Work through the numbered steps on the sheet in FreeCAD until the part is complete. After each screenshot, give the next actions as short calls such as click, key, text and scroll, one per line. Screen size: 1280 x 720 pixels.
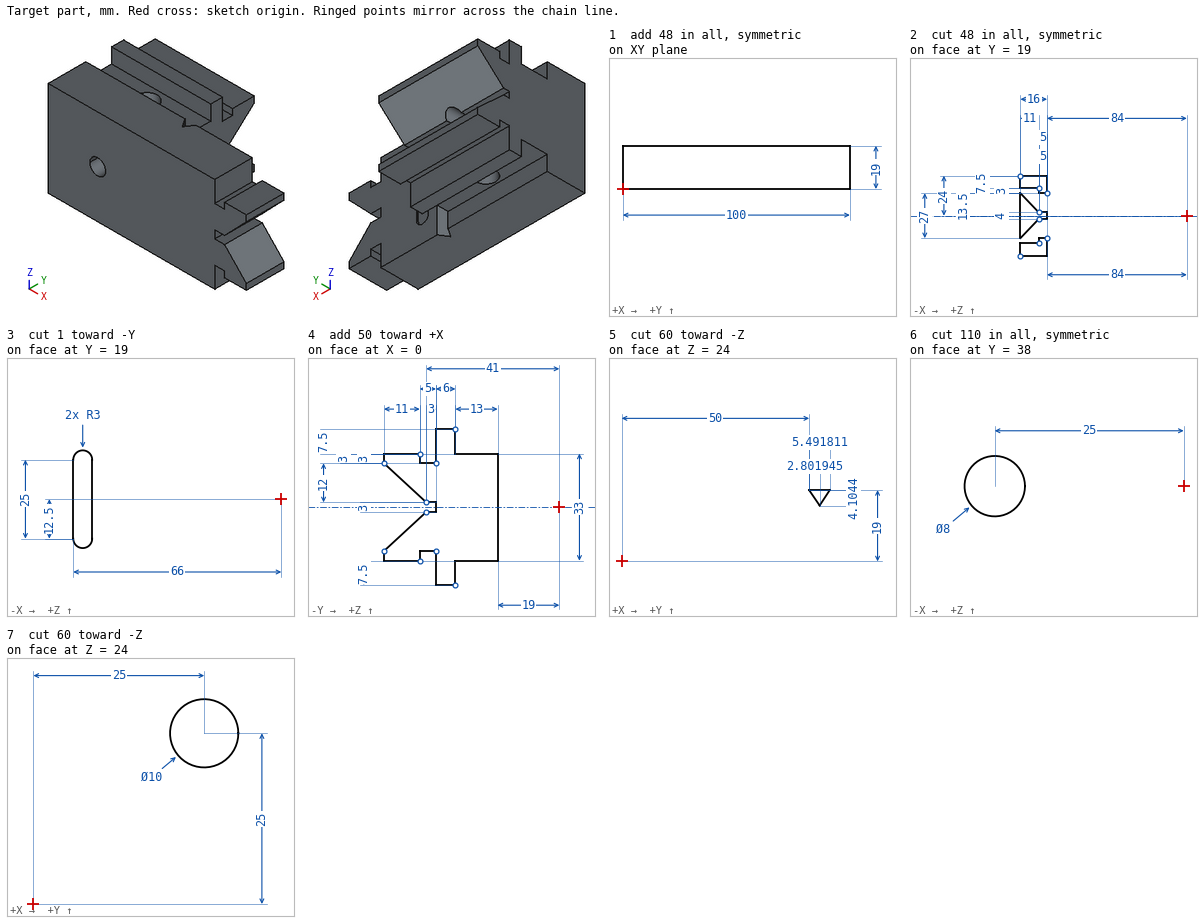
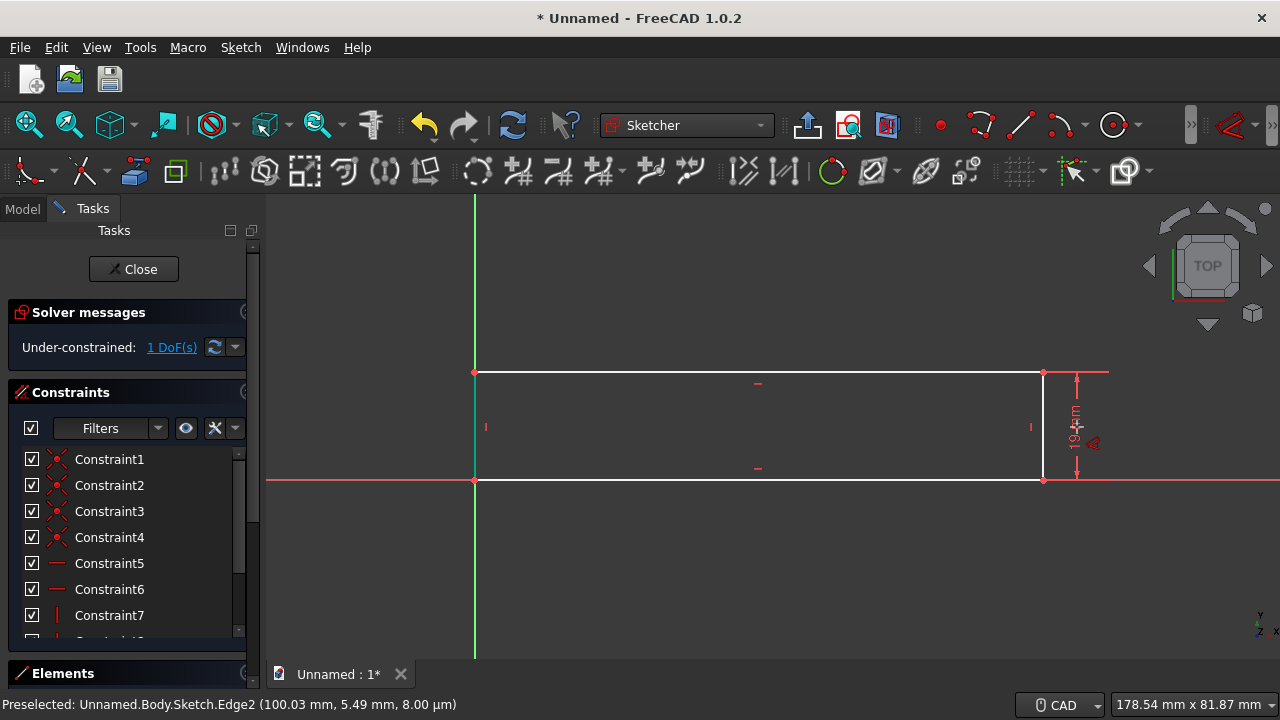
click(645, 480)
click(759, 514)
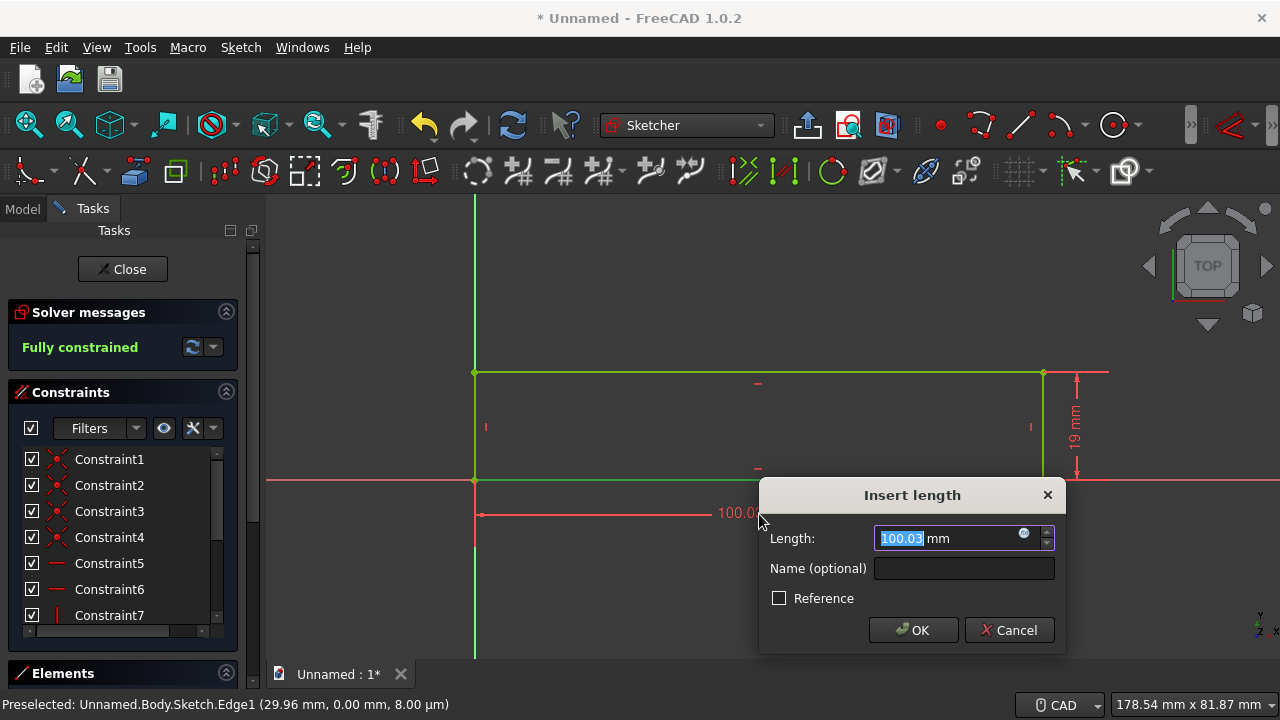
text(100)
key(Return)
key(Escape)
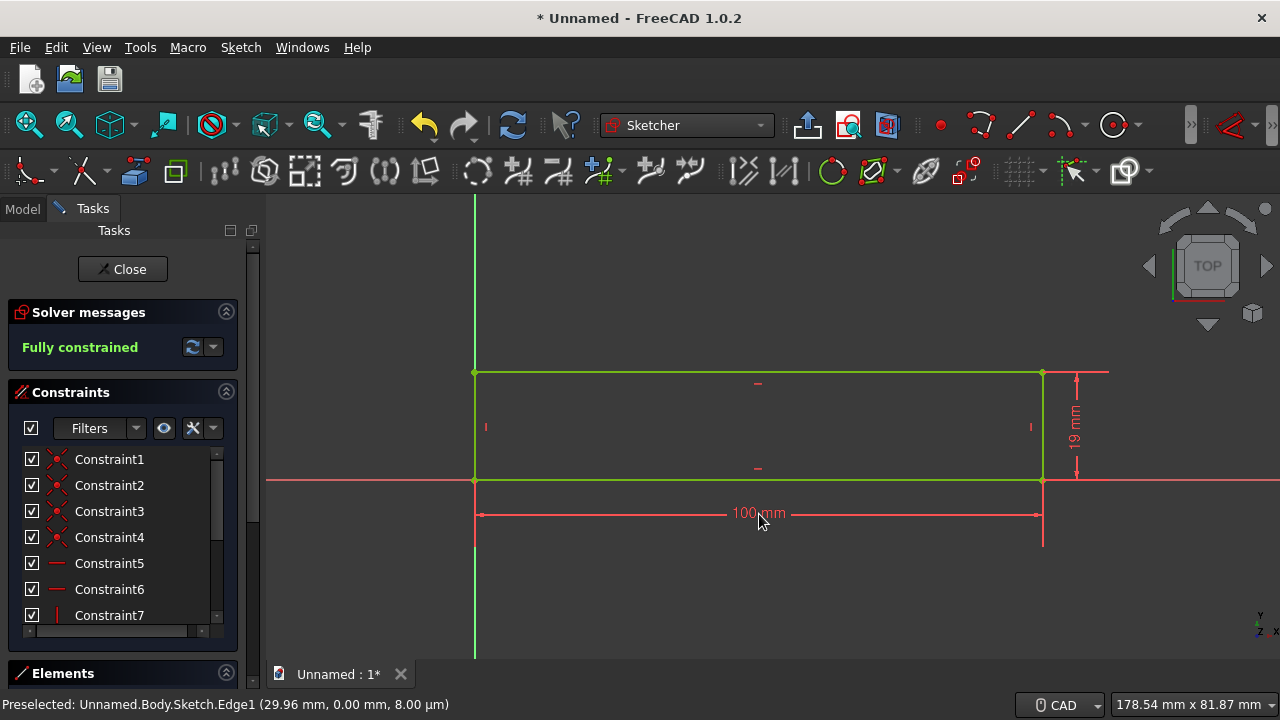
click(123, 269)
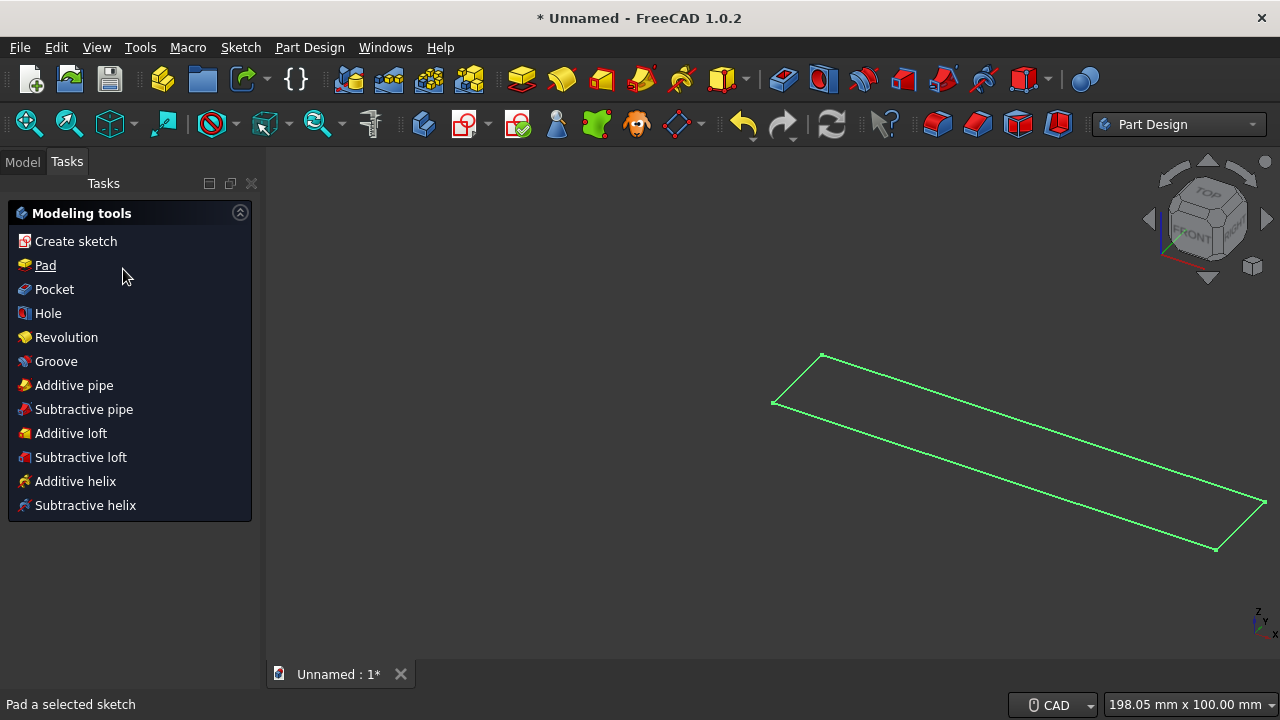
click(522, 80)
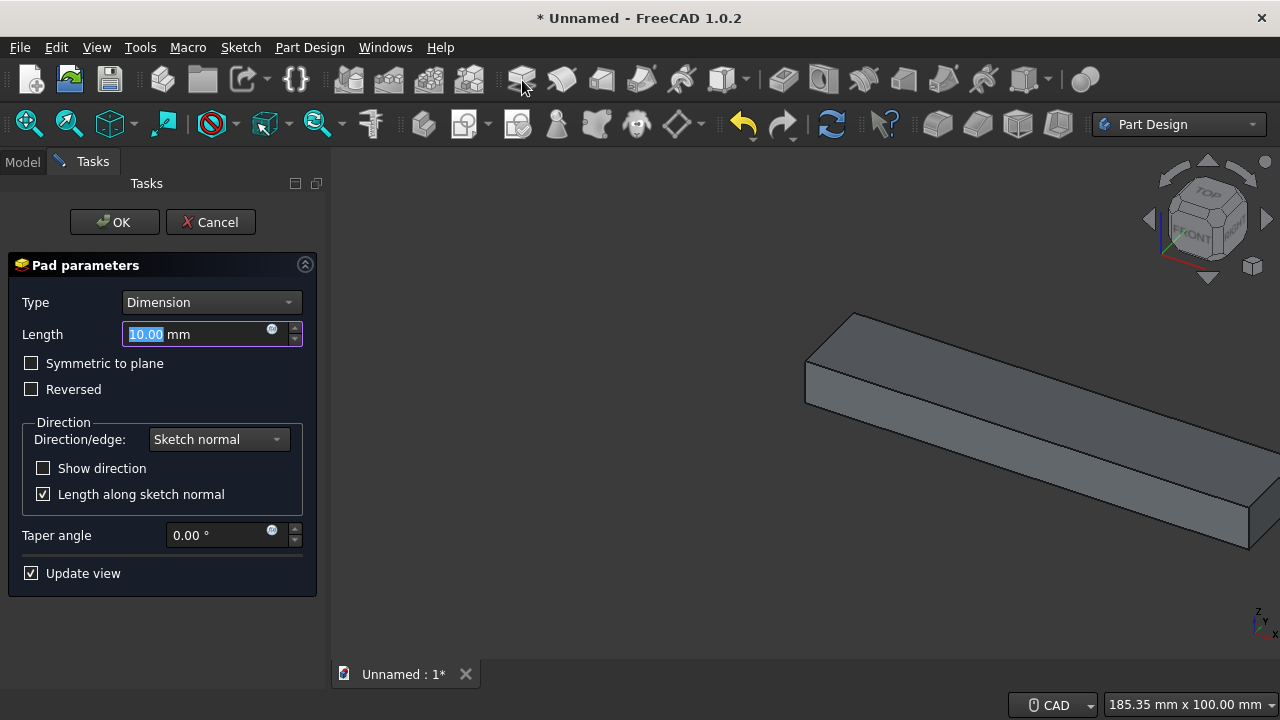
text(48)
key(Tab)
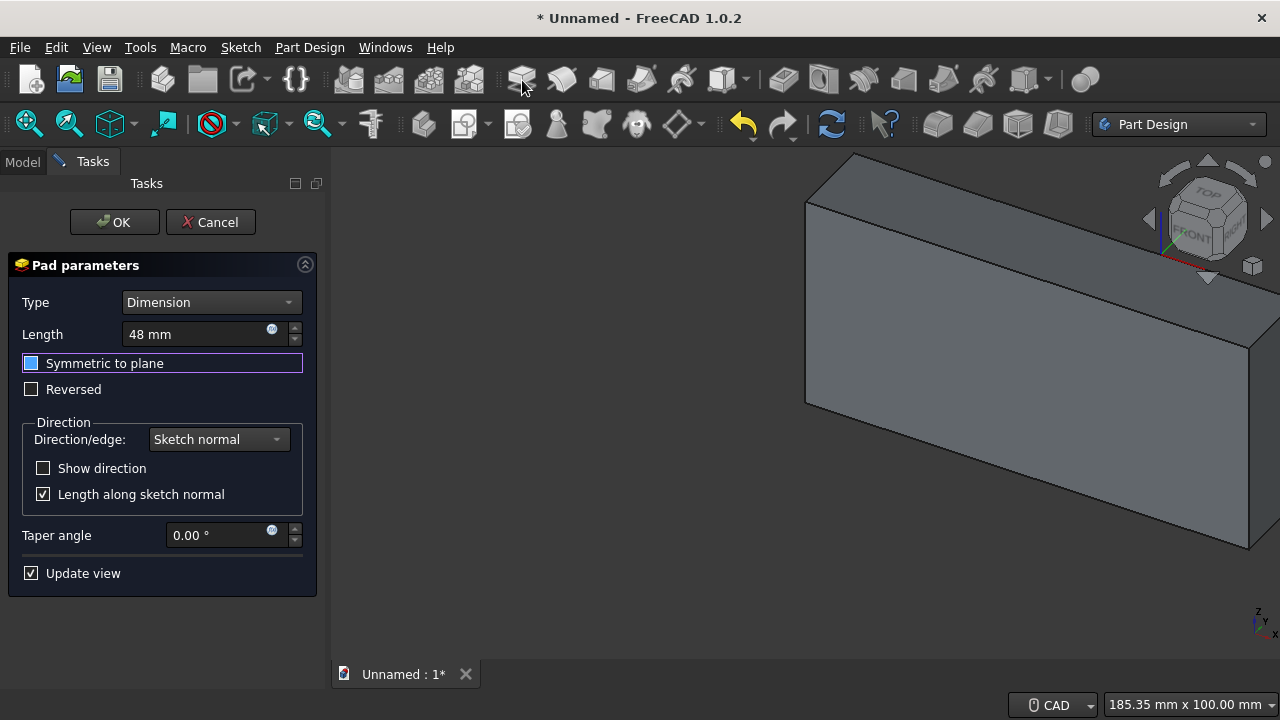
click(30, 363)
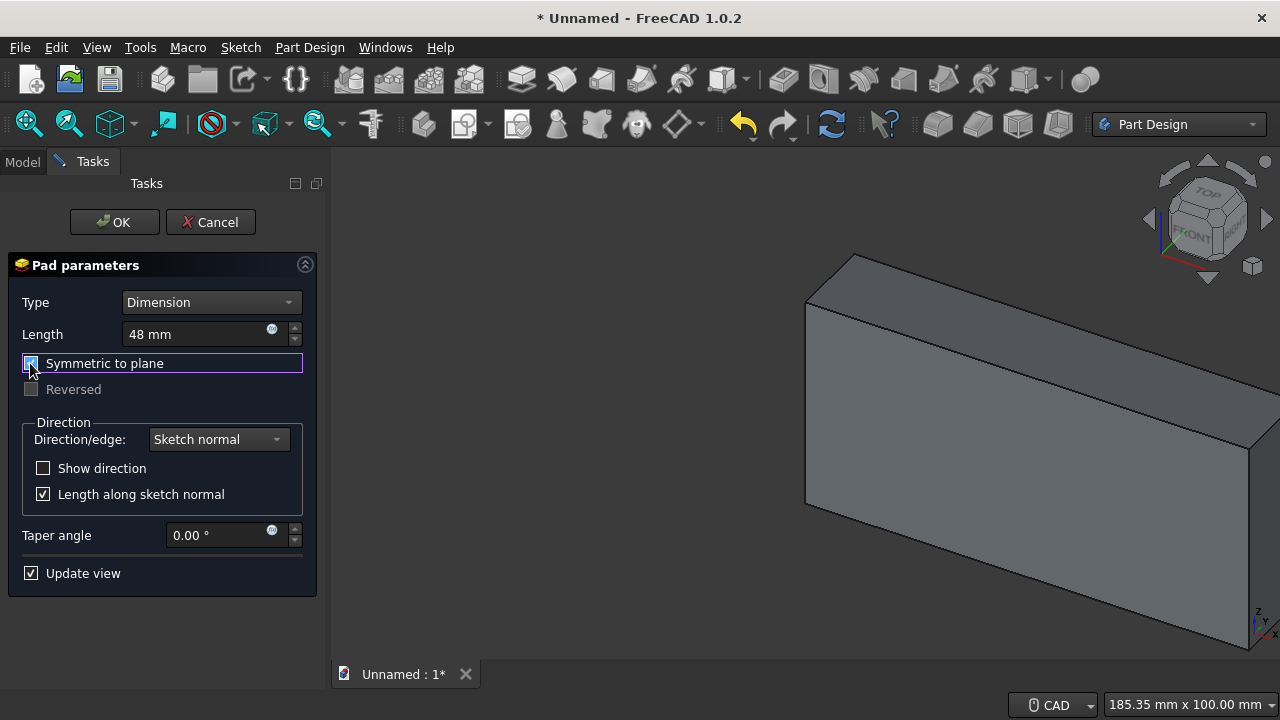
click(115, 222)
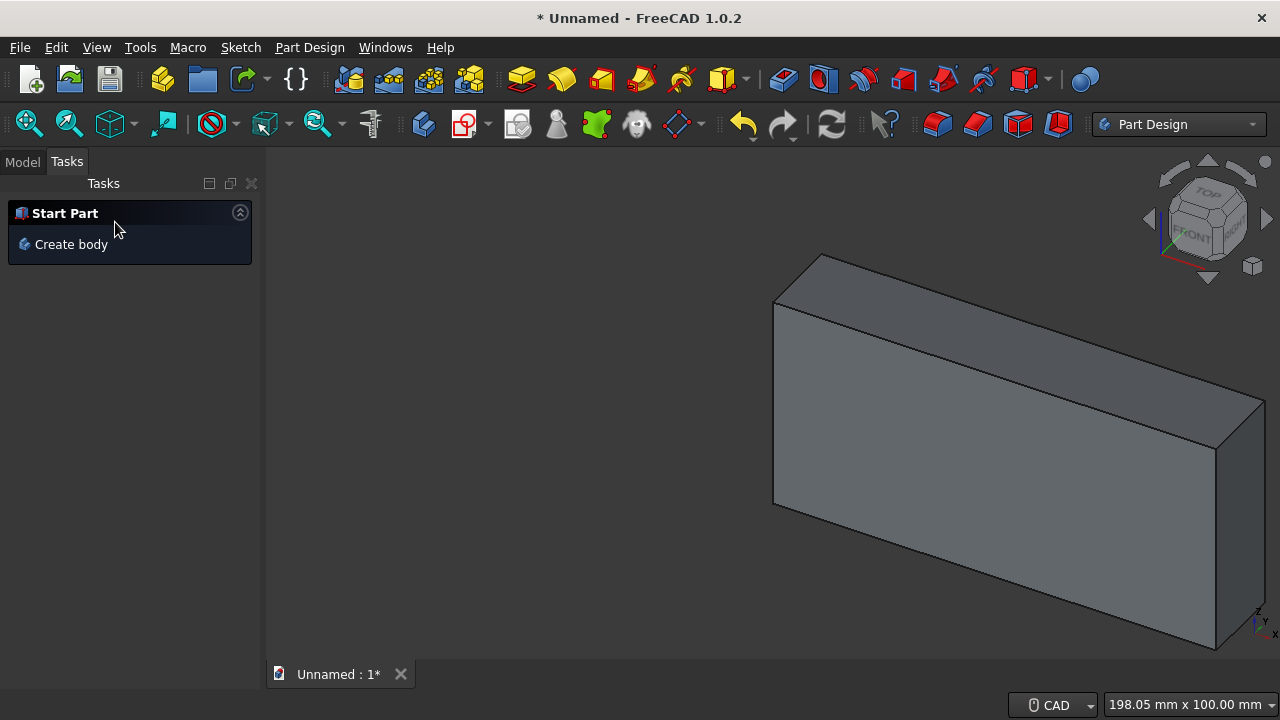
key(4)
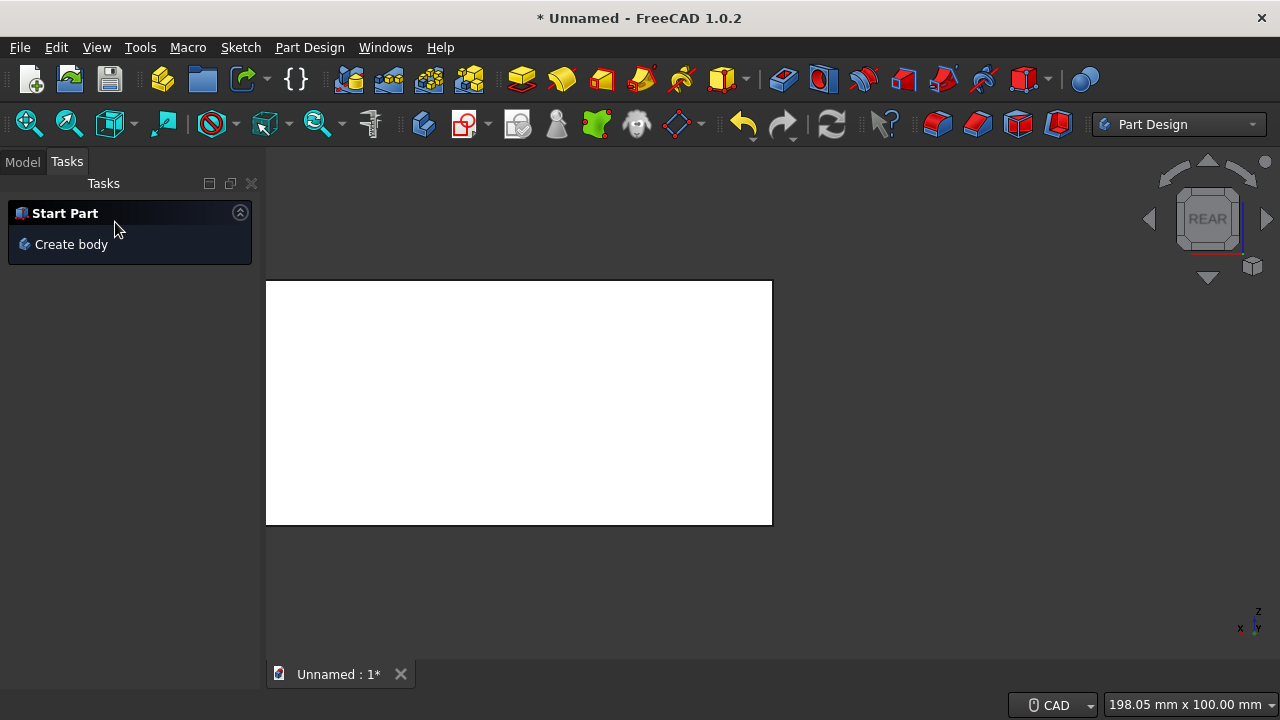
click(30, 124)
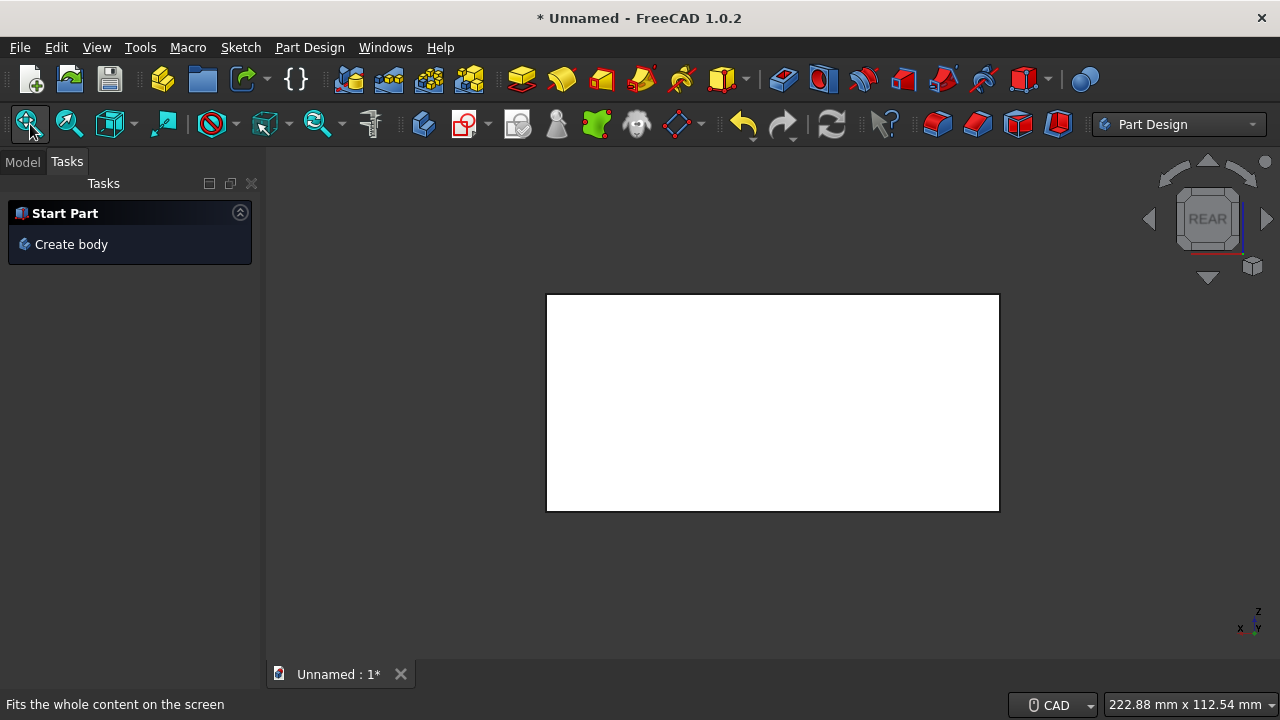
click(708, 402)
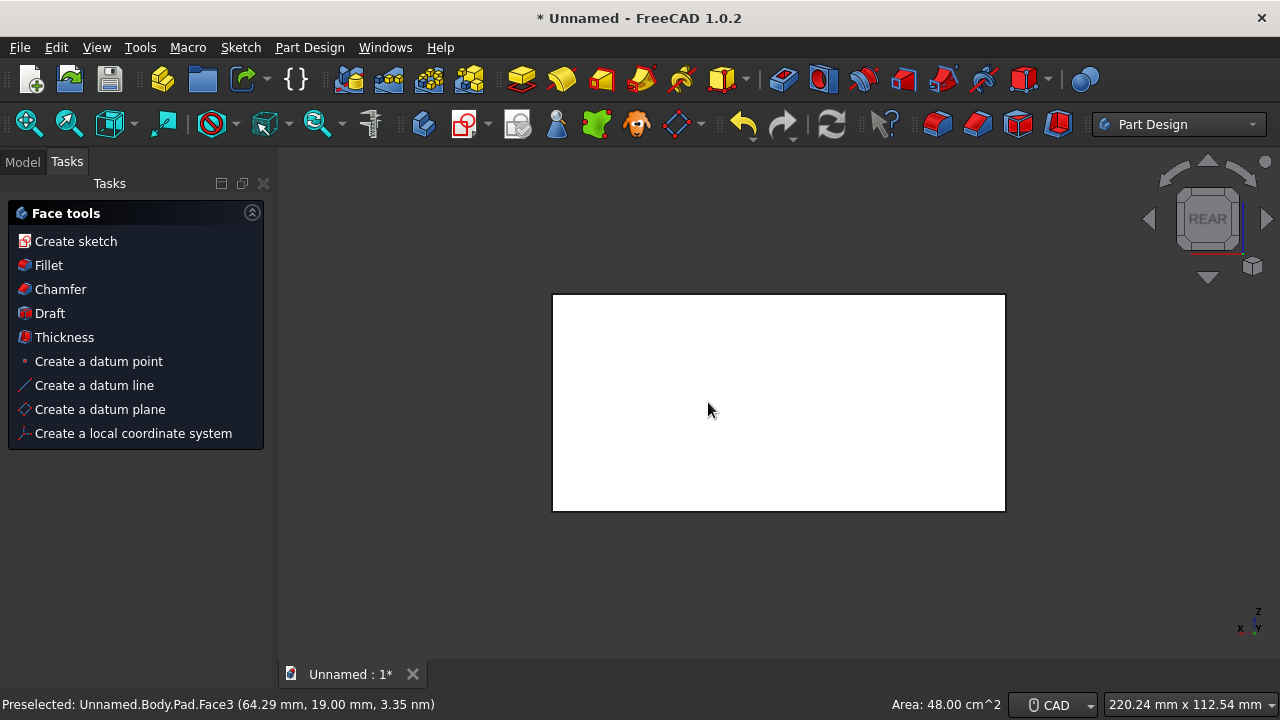
click(464, 124)